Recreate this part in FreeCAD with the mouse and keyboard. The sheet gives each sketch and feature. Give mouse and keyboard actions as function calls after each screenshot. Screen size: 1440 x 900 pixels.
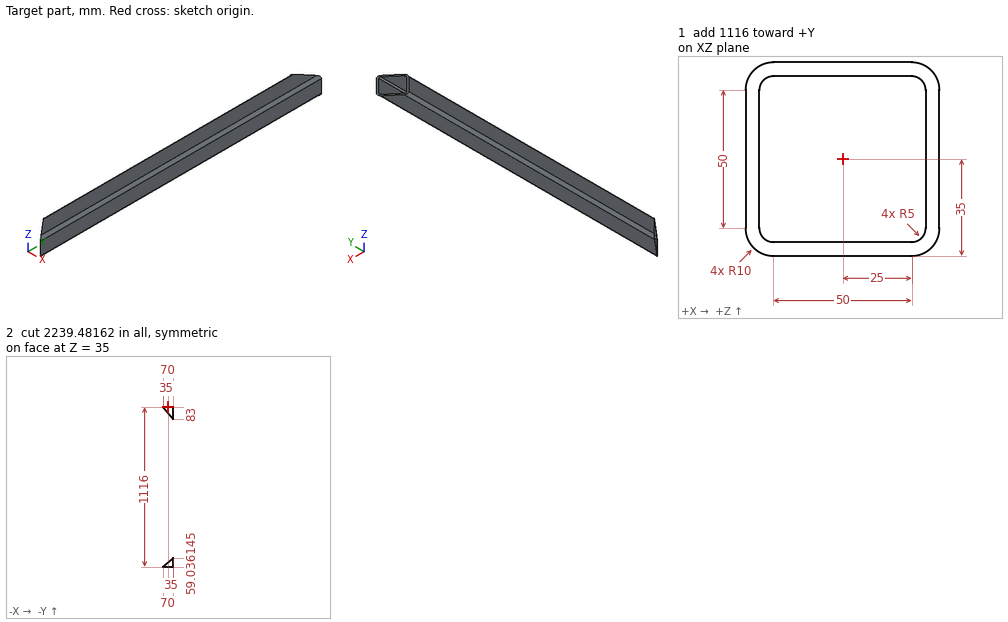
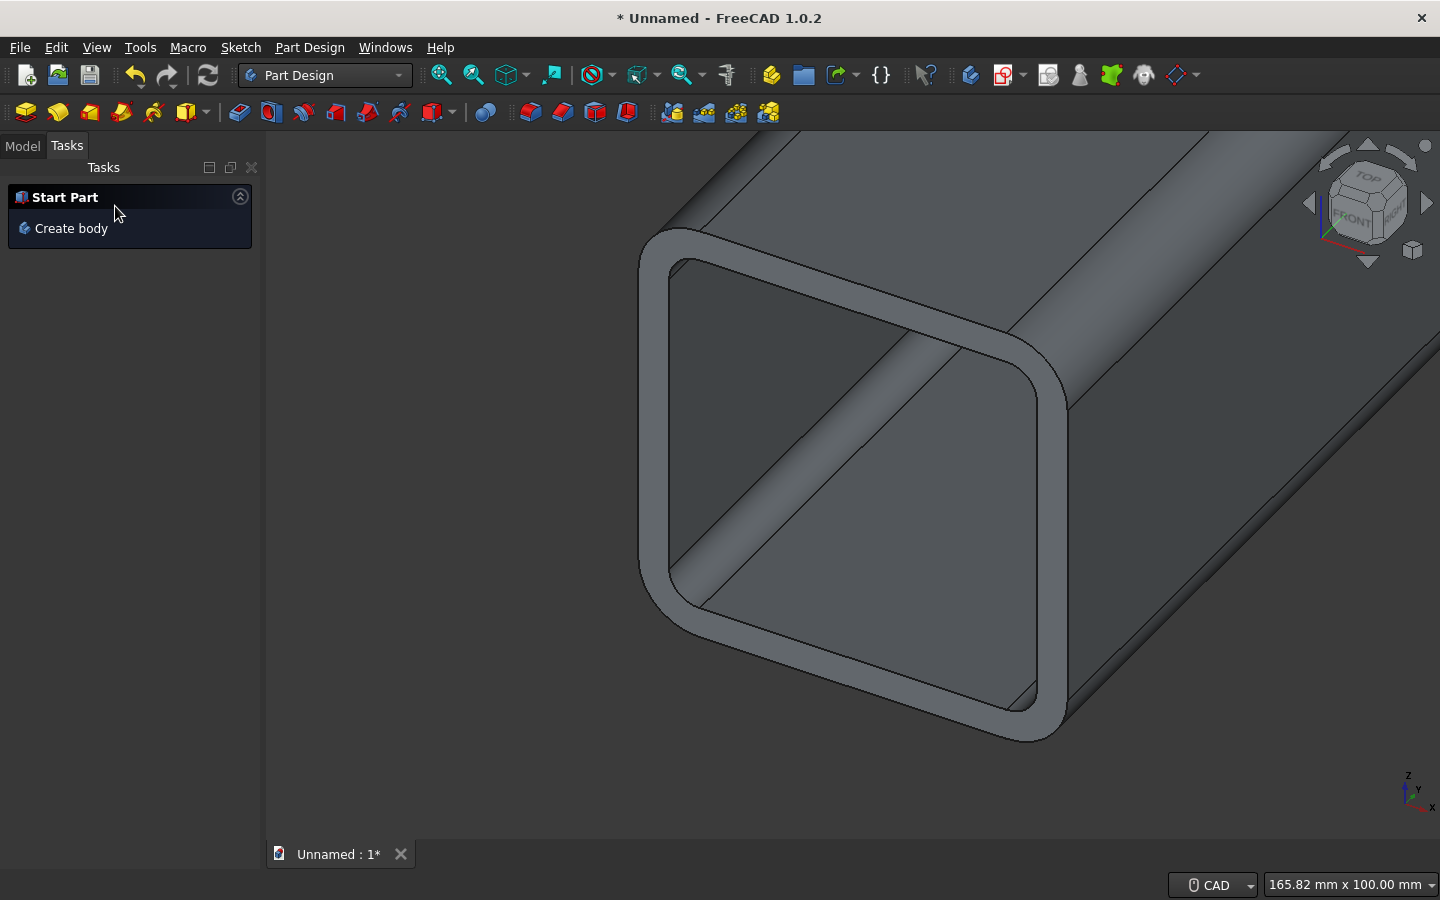
key(v)
key(f)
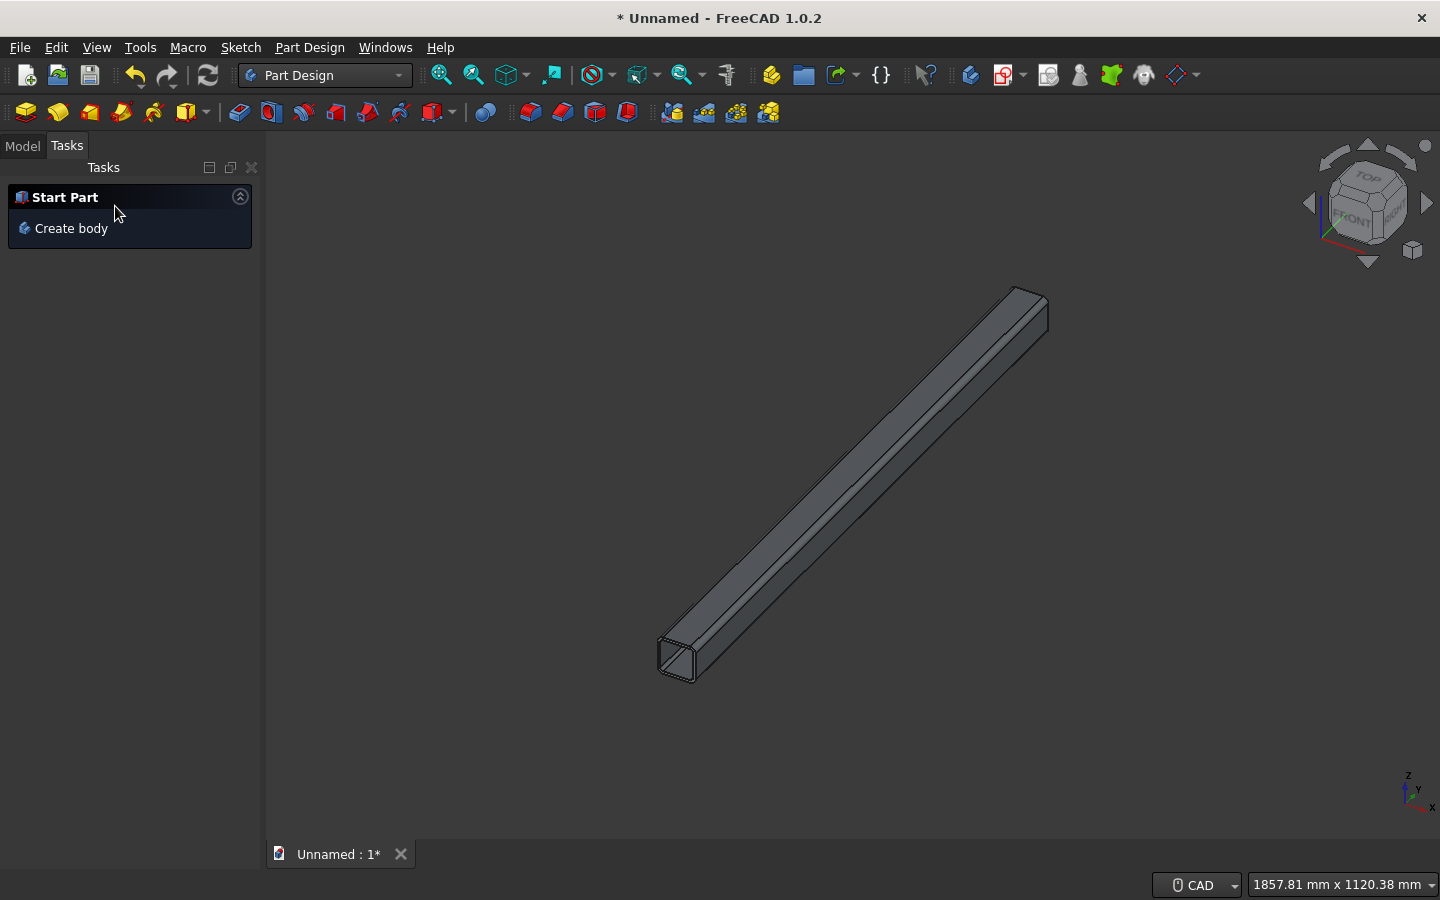
click(1004, 316)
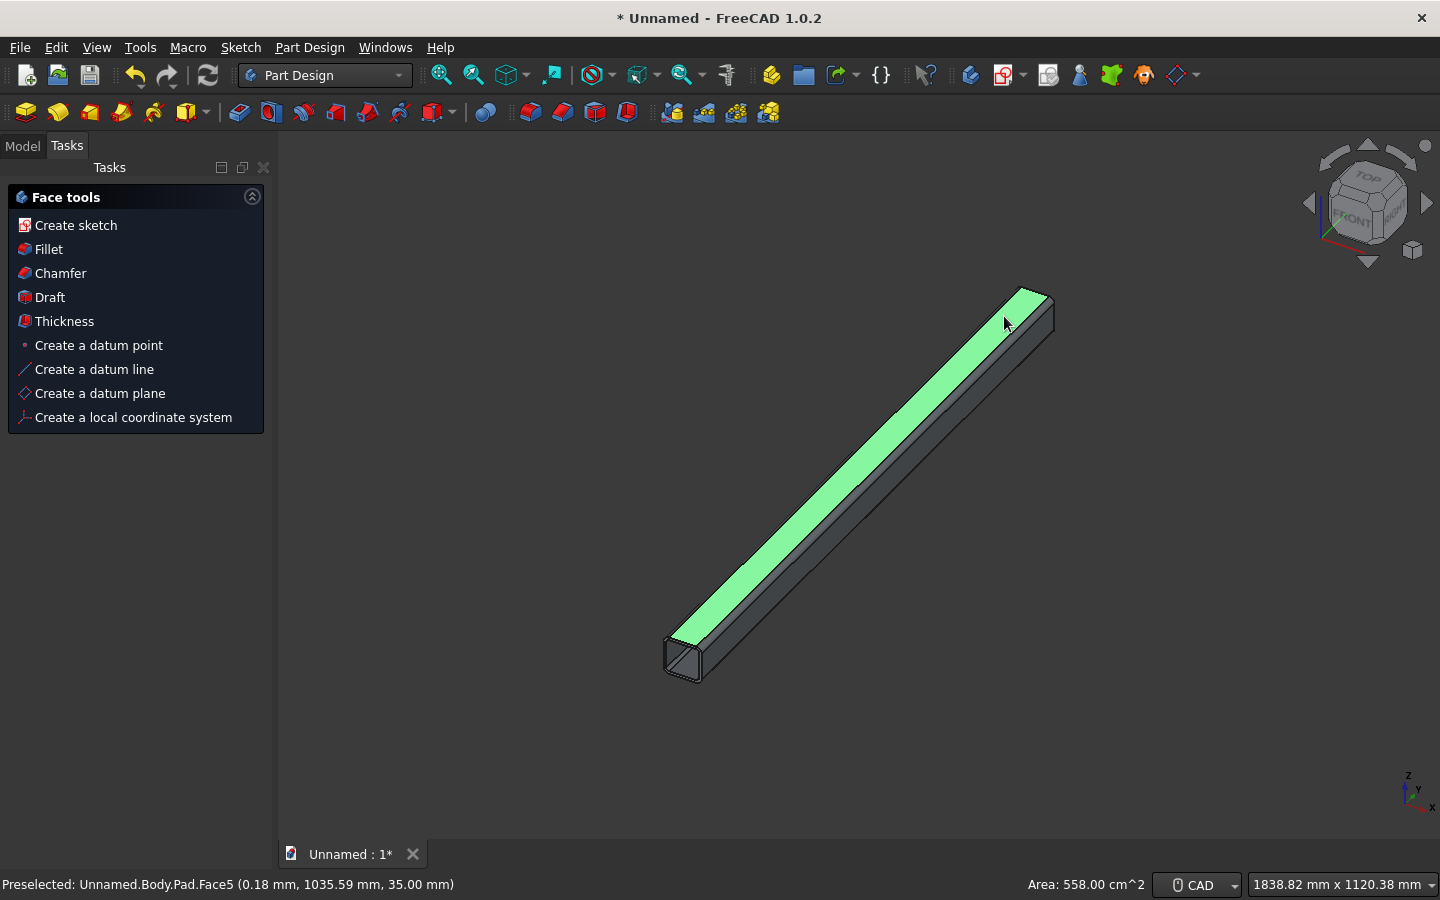
click(1004, 76)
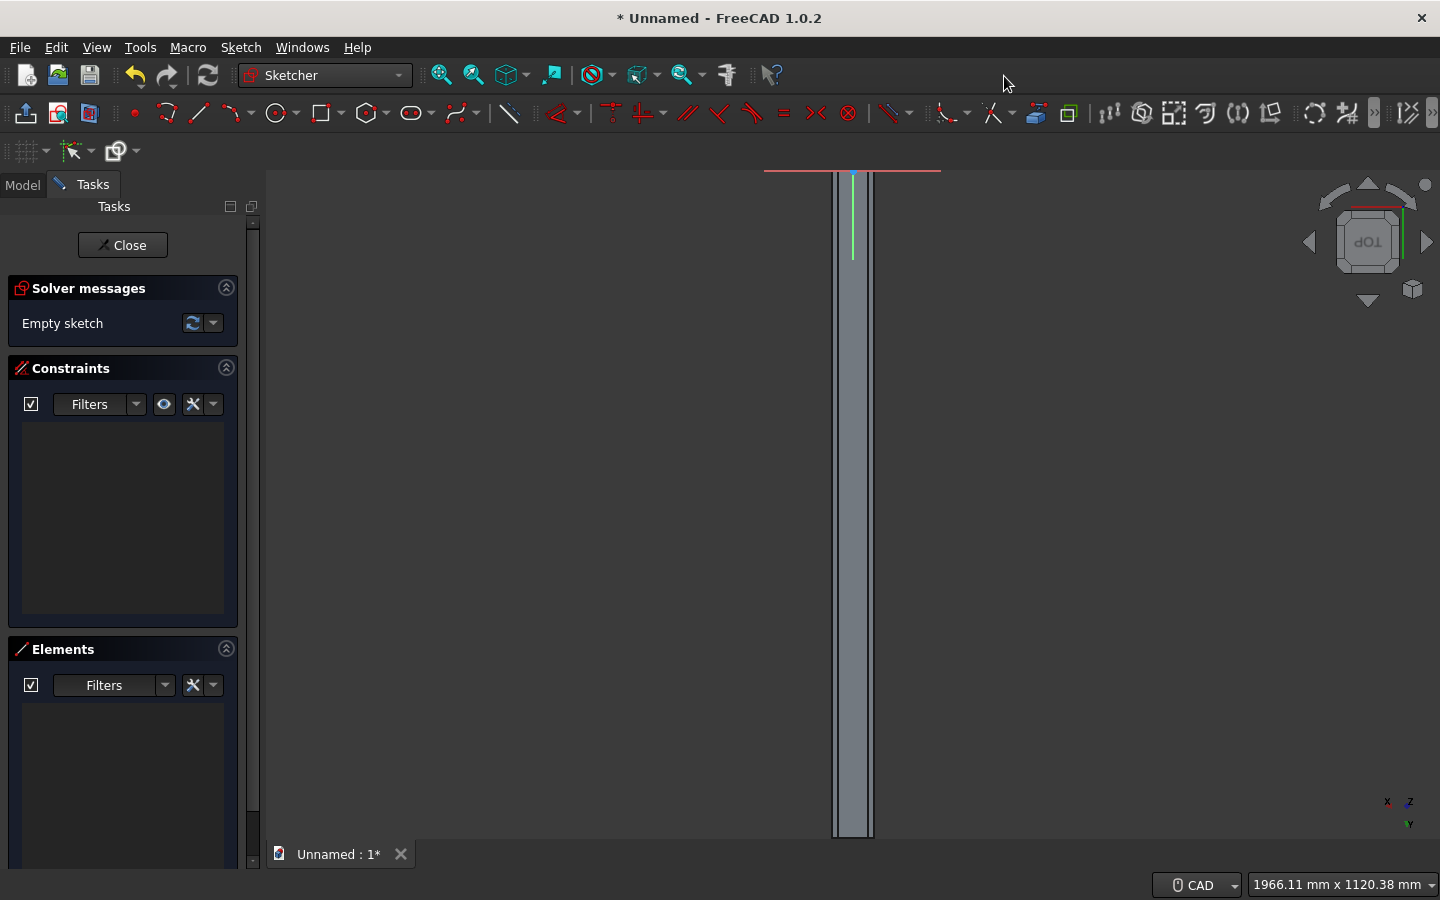
scroll(645, 505, down, 2)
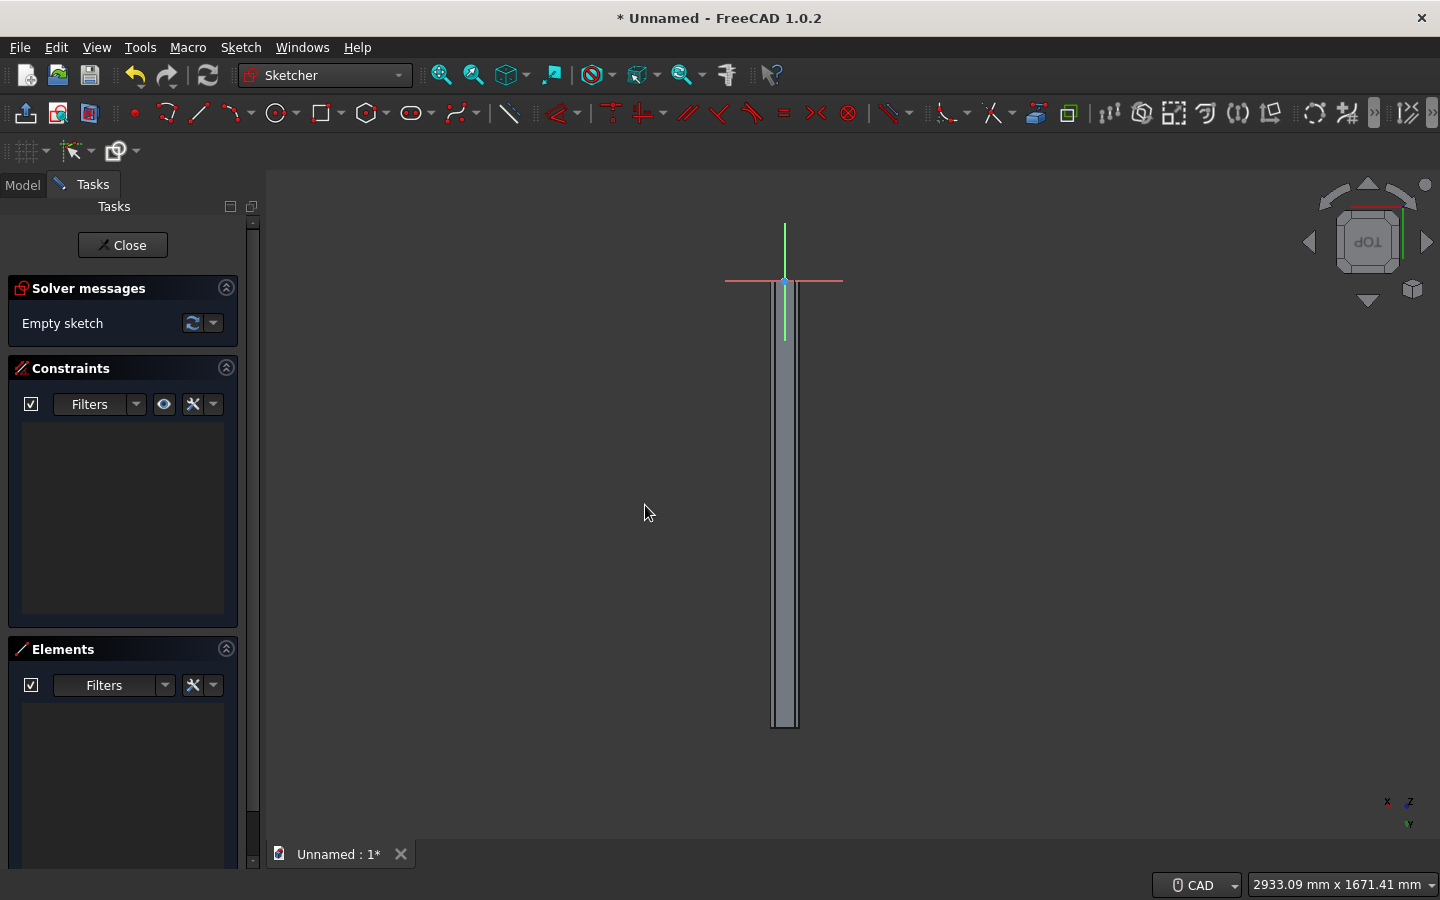
key(g)
key(m)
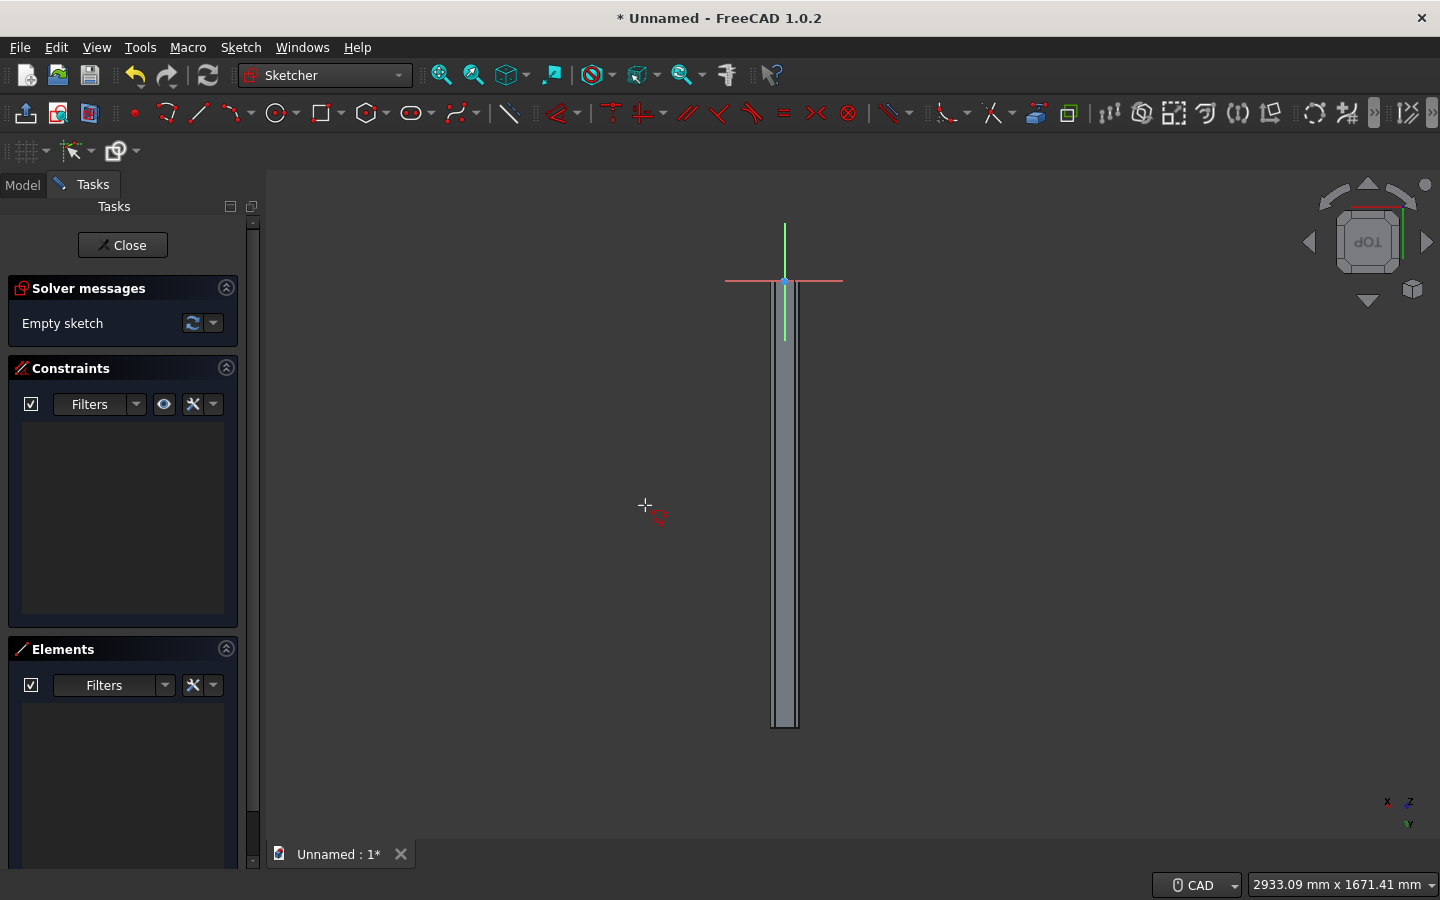
click(799, 705)
click(771, 728)
click(799, 728)
click(799, 706)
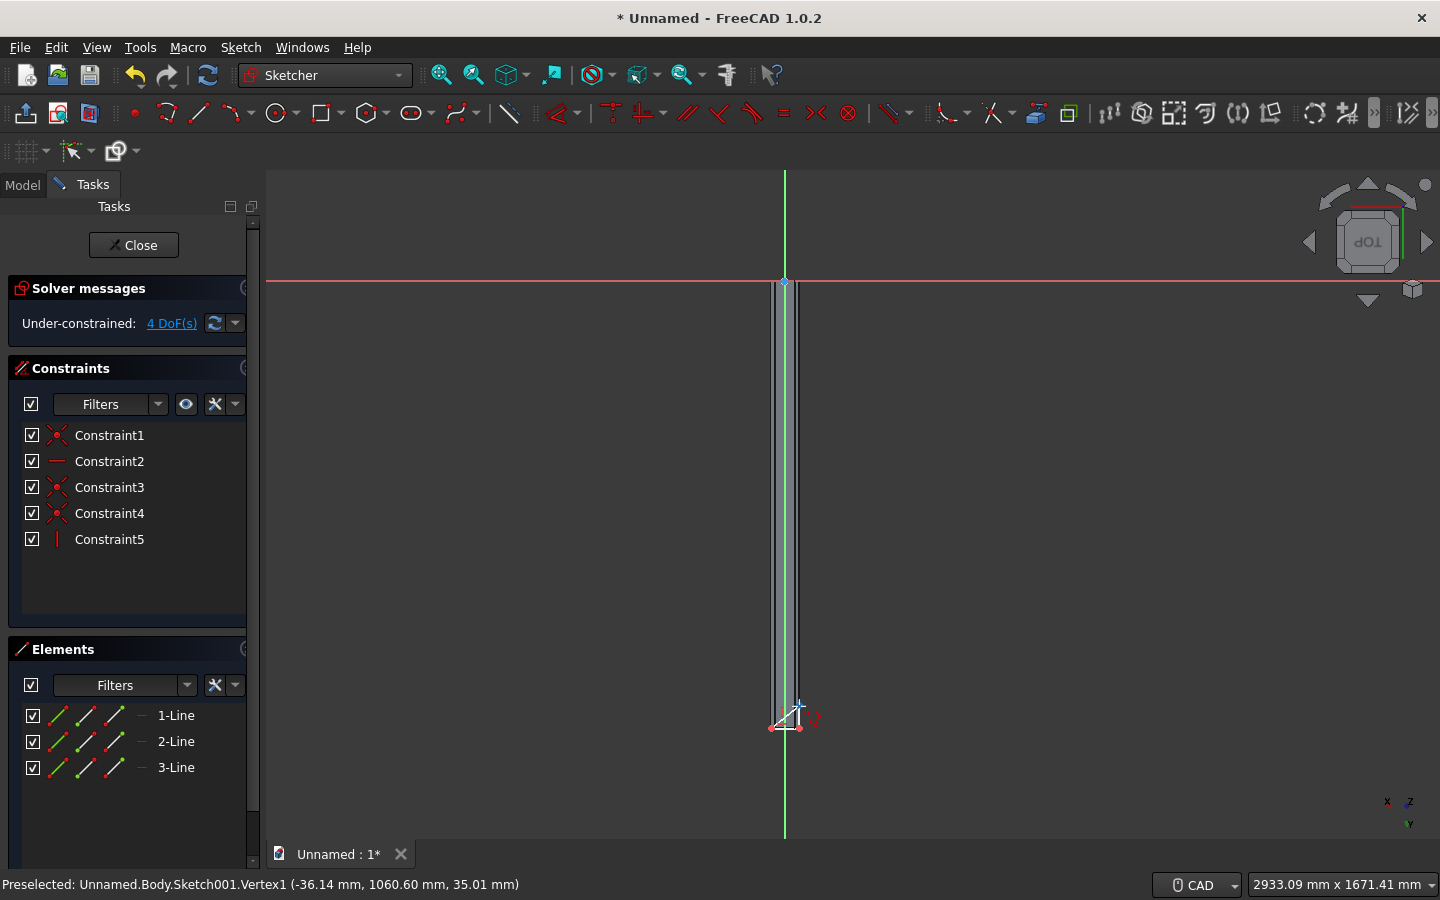
click(771, 281)
click(799, 315)
click(799, 290)
click(771, 281)
key(Escape)
key(Escape)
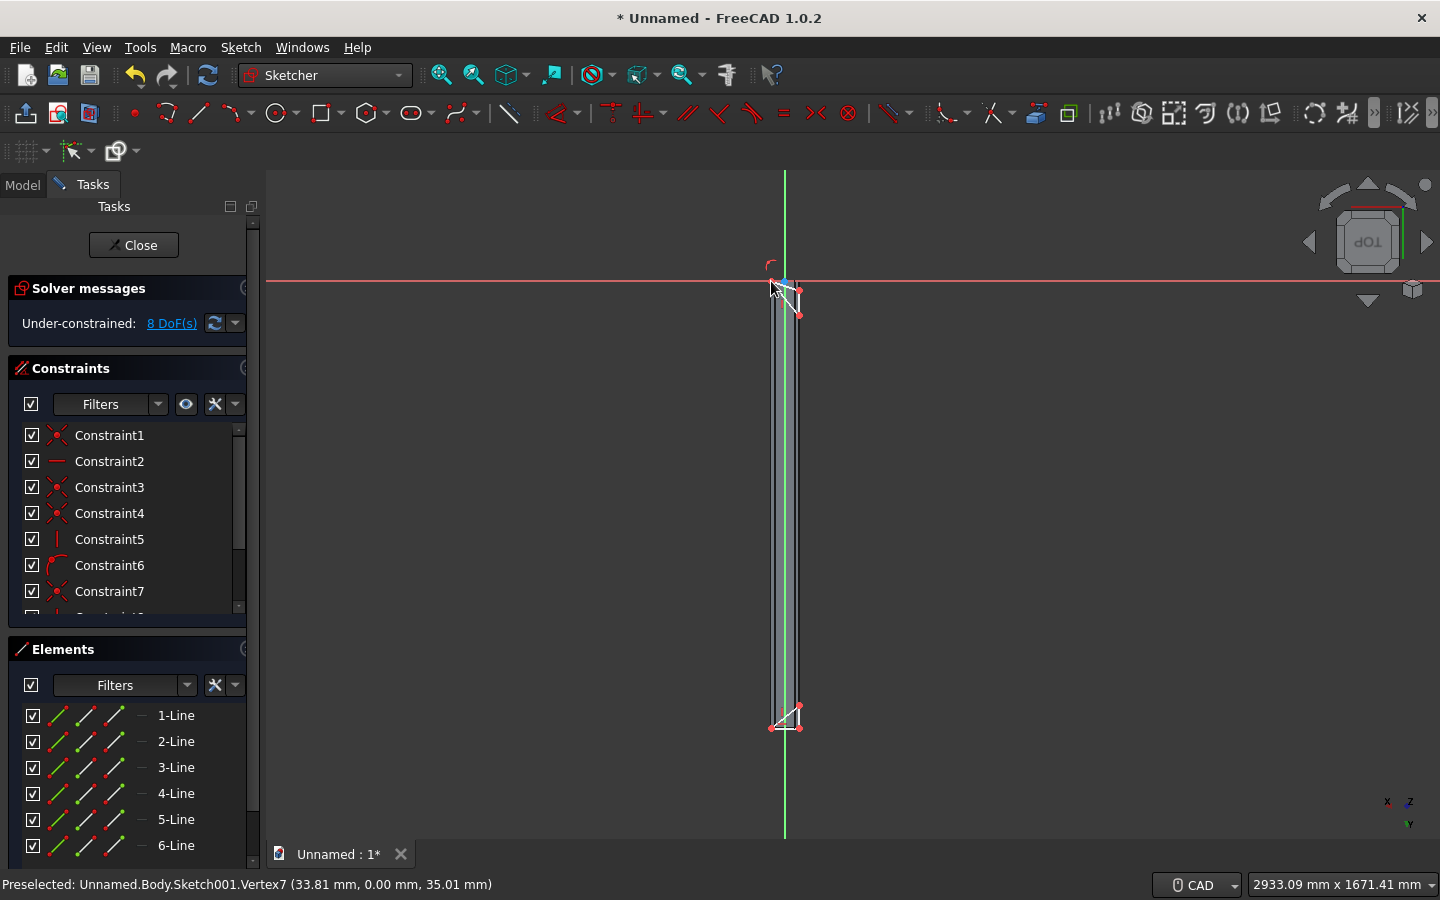
scroll(782, 285, up, 4)